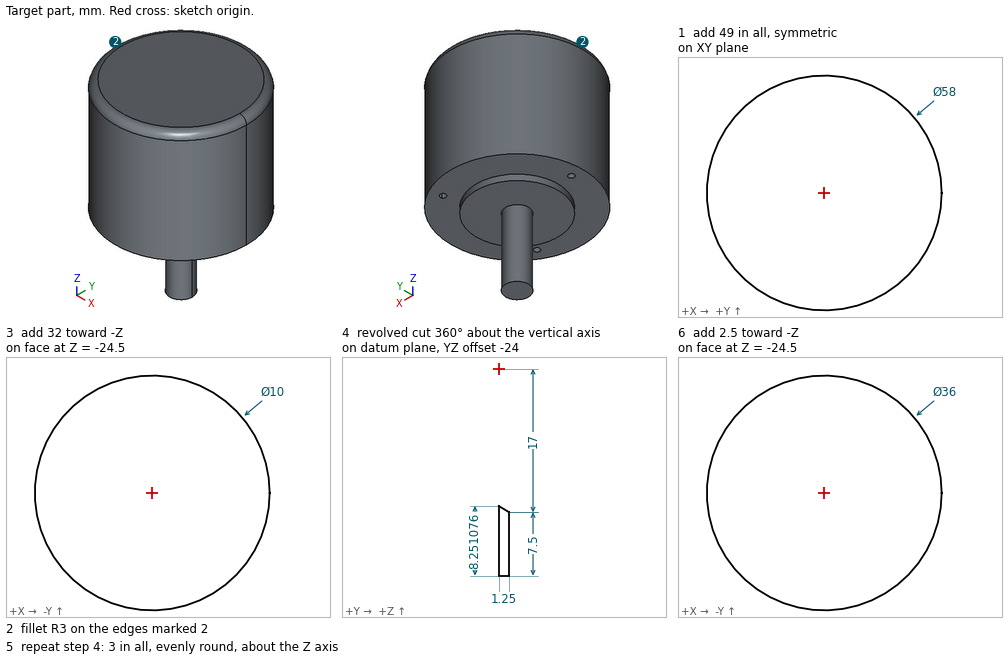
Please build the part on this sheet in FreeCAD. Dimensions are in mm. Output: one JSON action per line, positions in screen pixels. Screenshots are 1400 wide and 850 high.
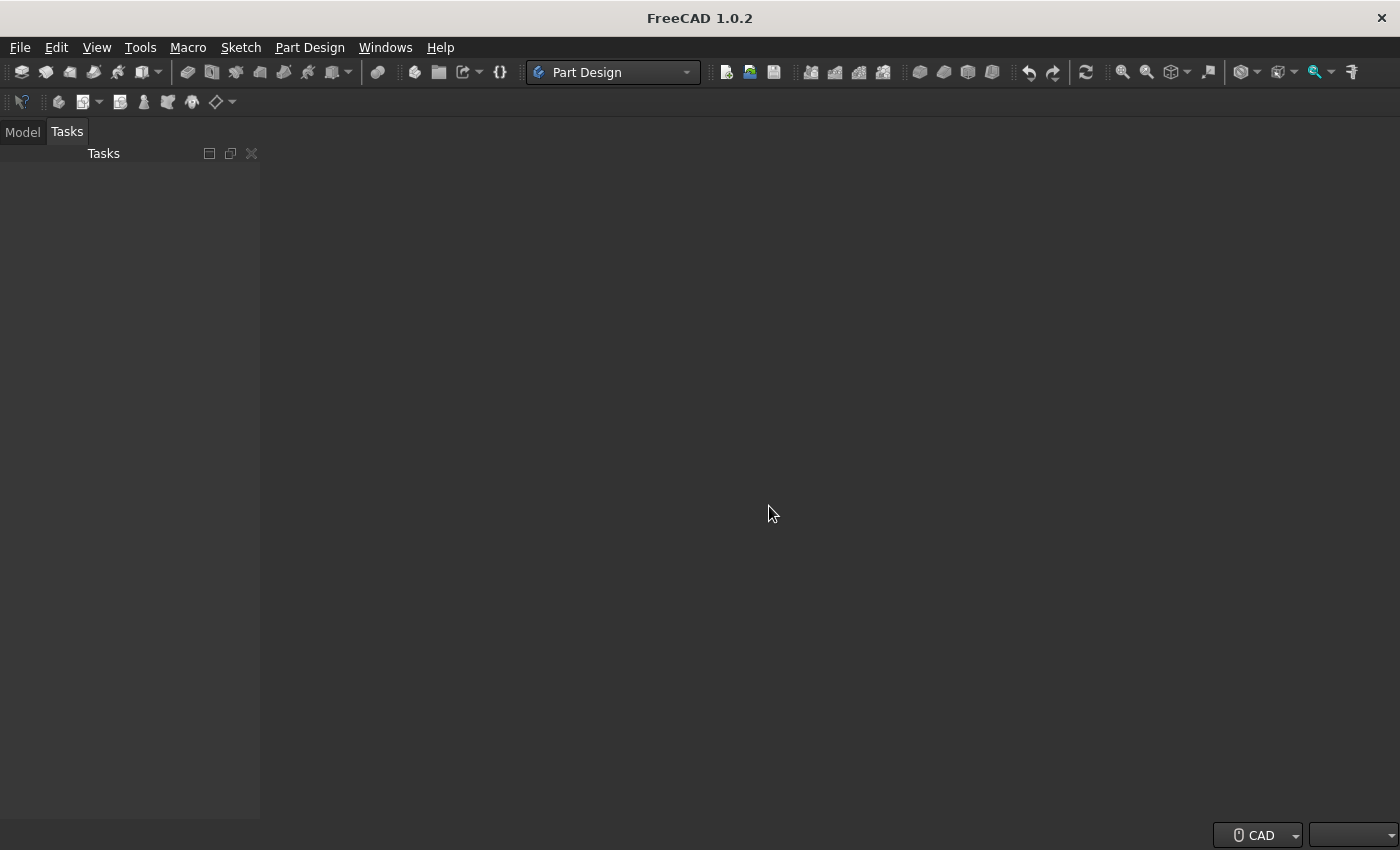
{"action": "left_click", "coordinate": [726, 72]}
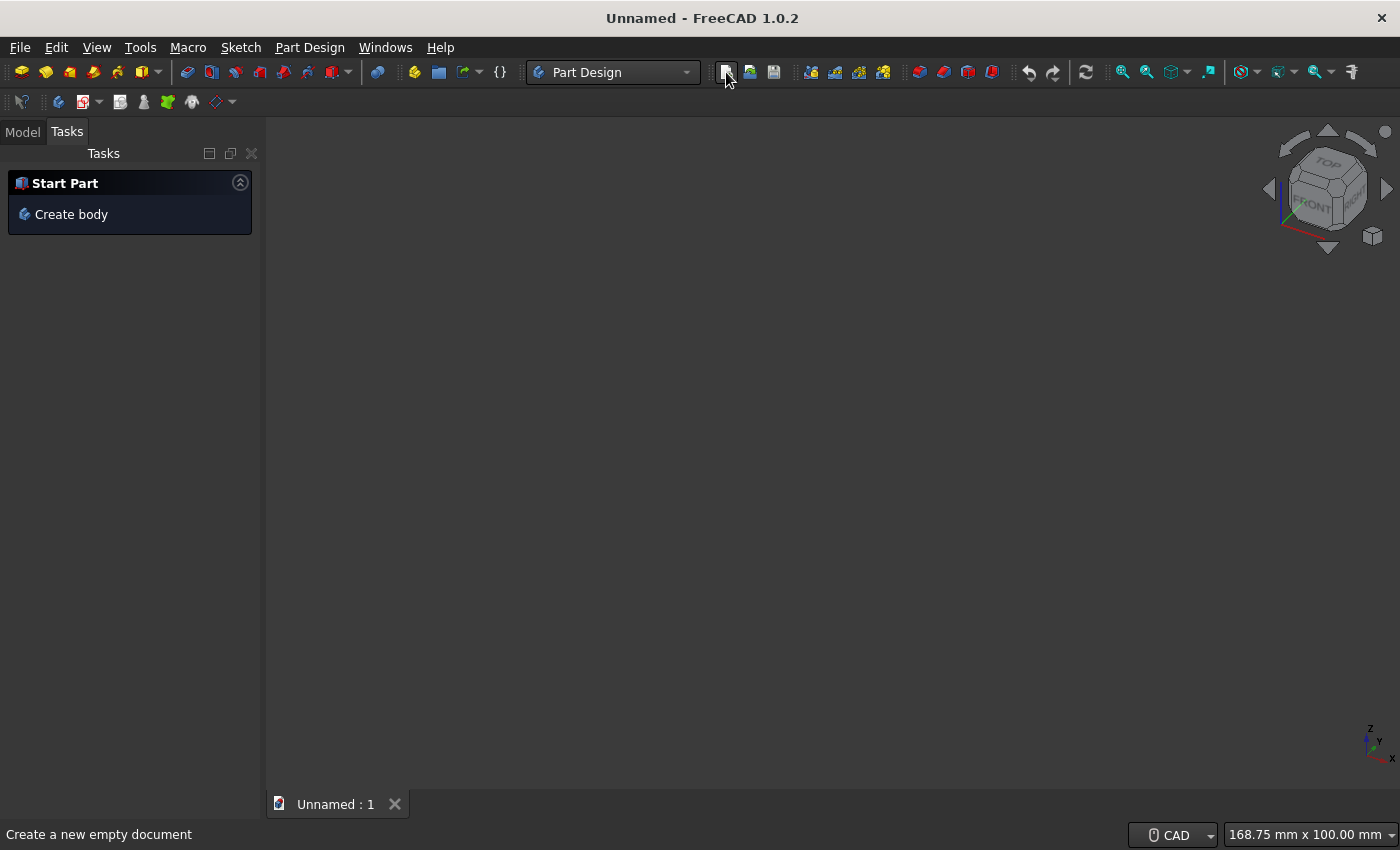
{"action": "left_click", "coordinate": [84, 102]}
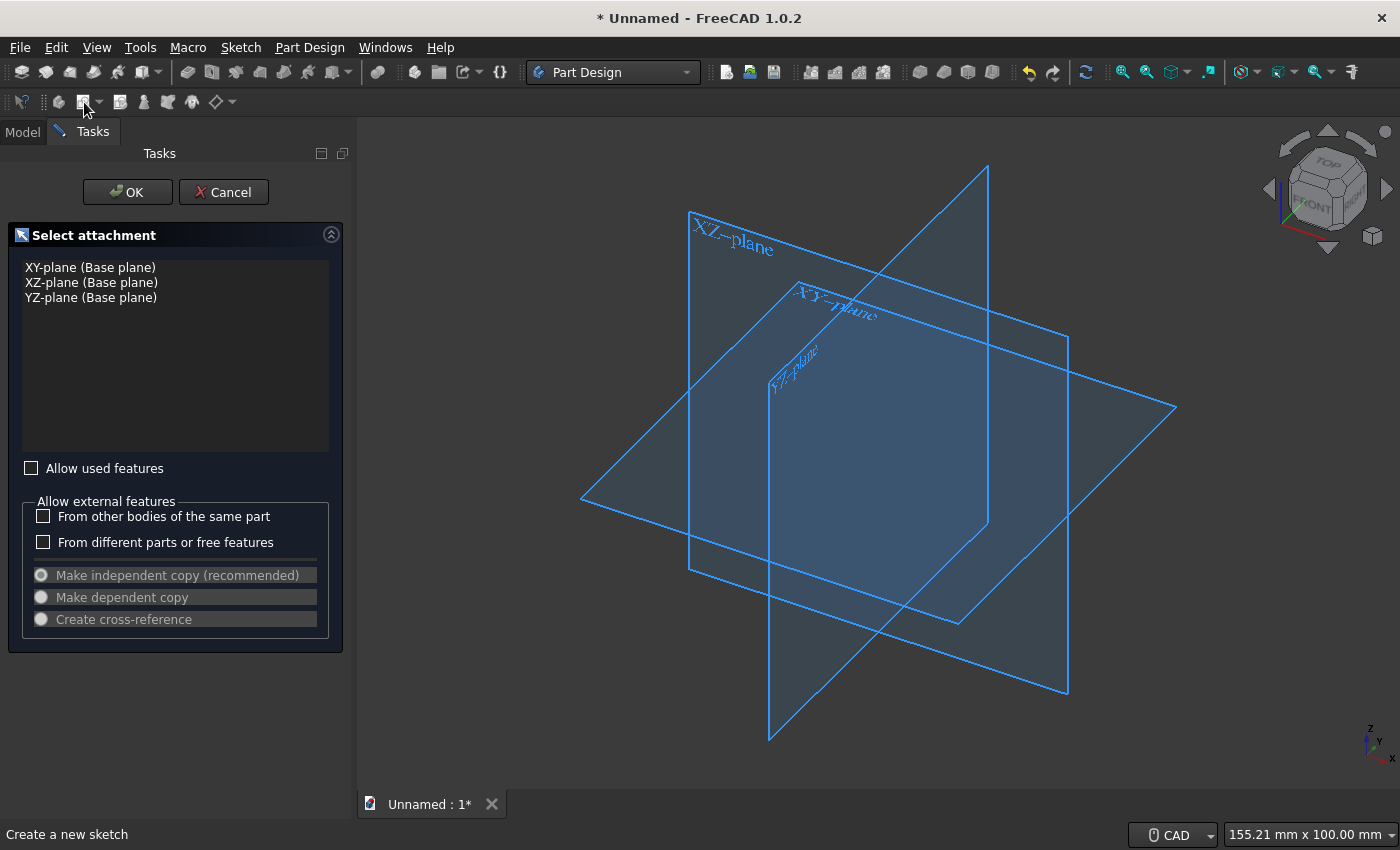
{"action": "left_click", "coordinate": [82, 268]}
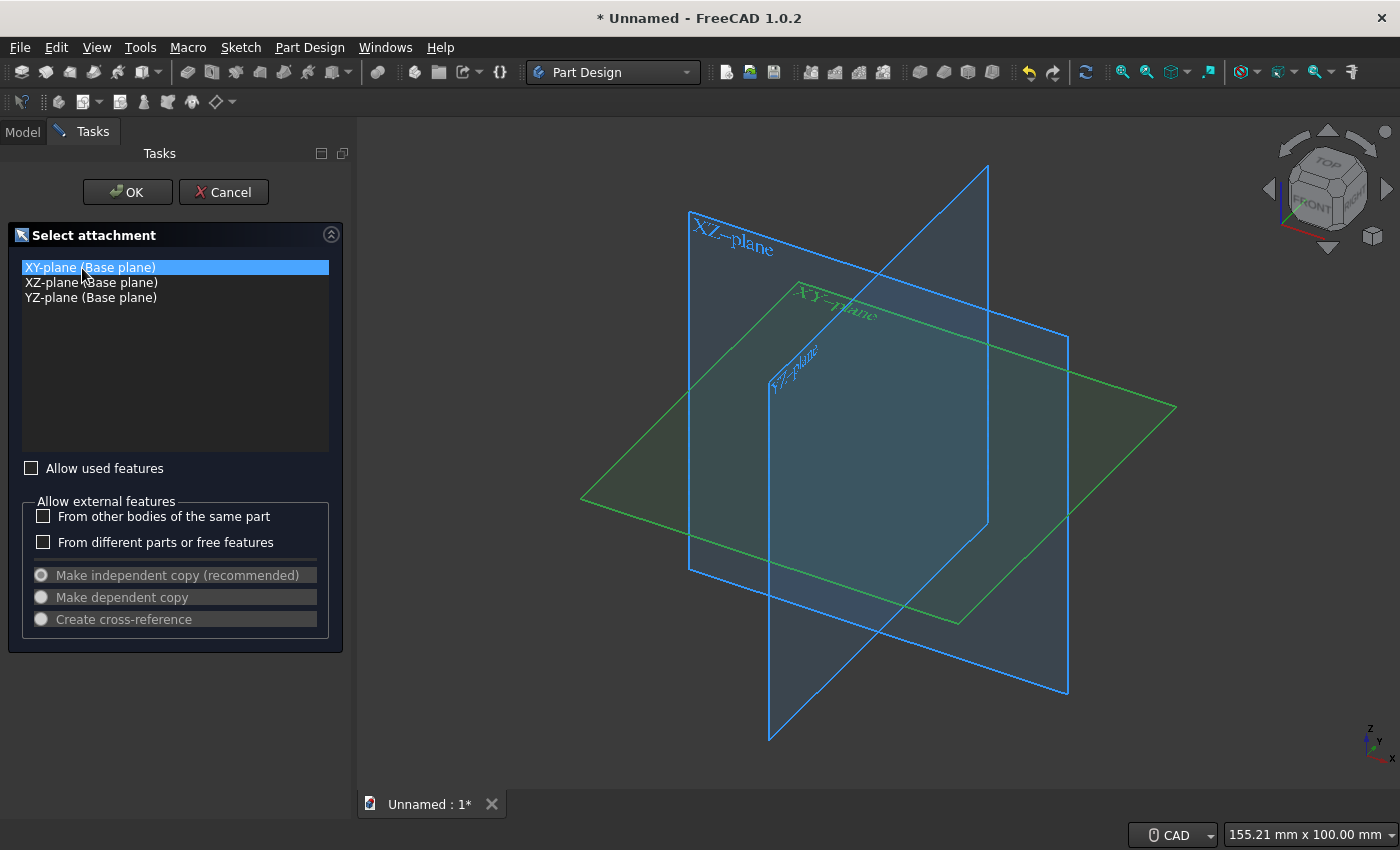
{"action": "left_click", "coordinate": [128, 192]}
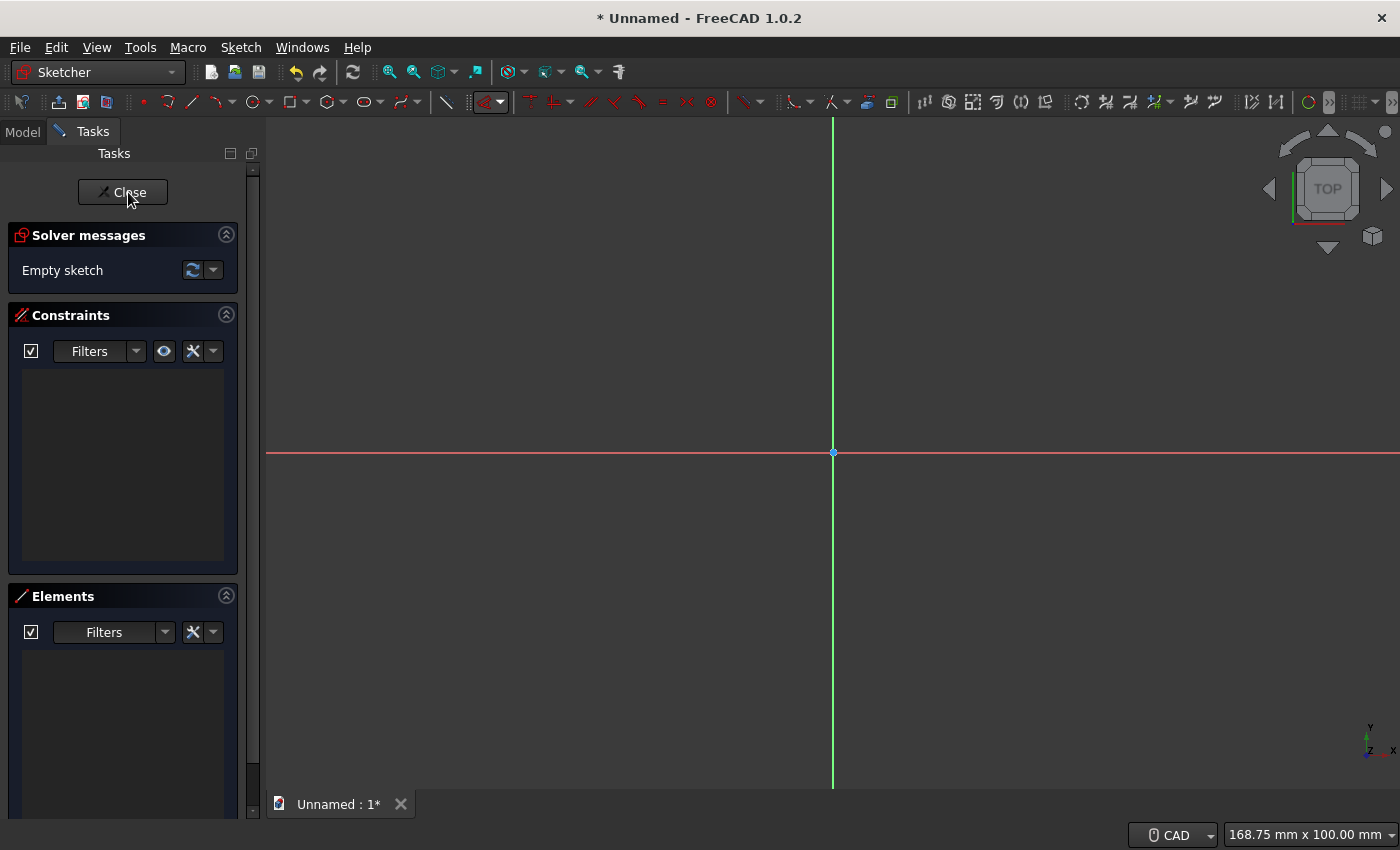
{"action": "left_click", "coordinate": [254, 102]}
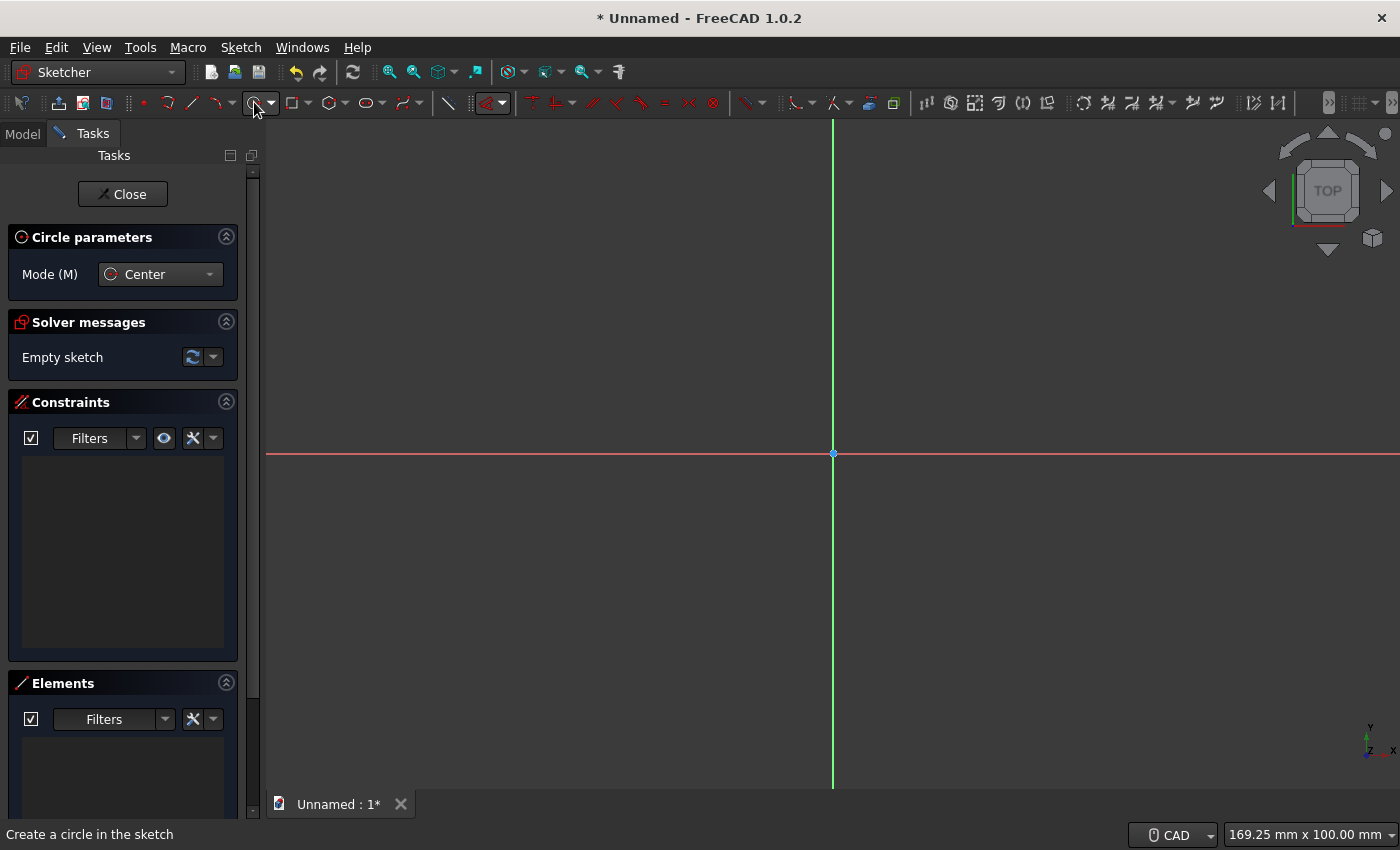
{"action": "left_click", "coordinate": [833, 454]}
{"action": "left_click", "coordinate": [970, 317]}
{"action": "key", "text": "Escape"}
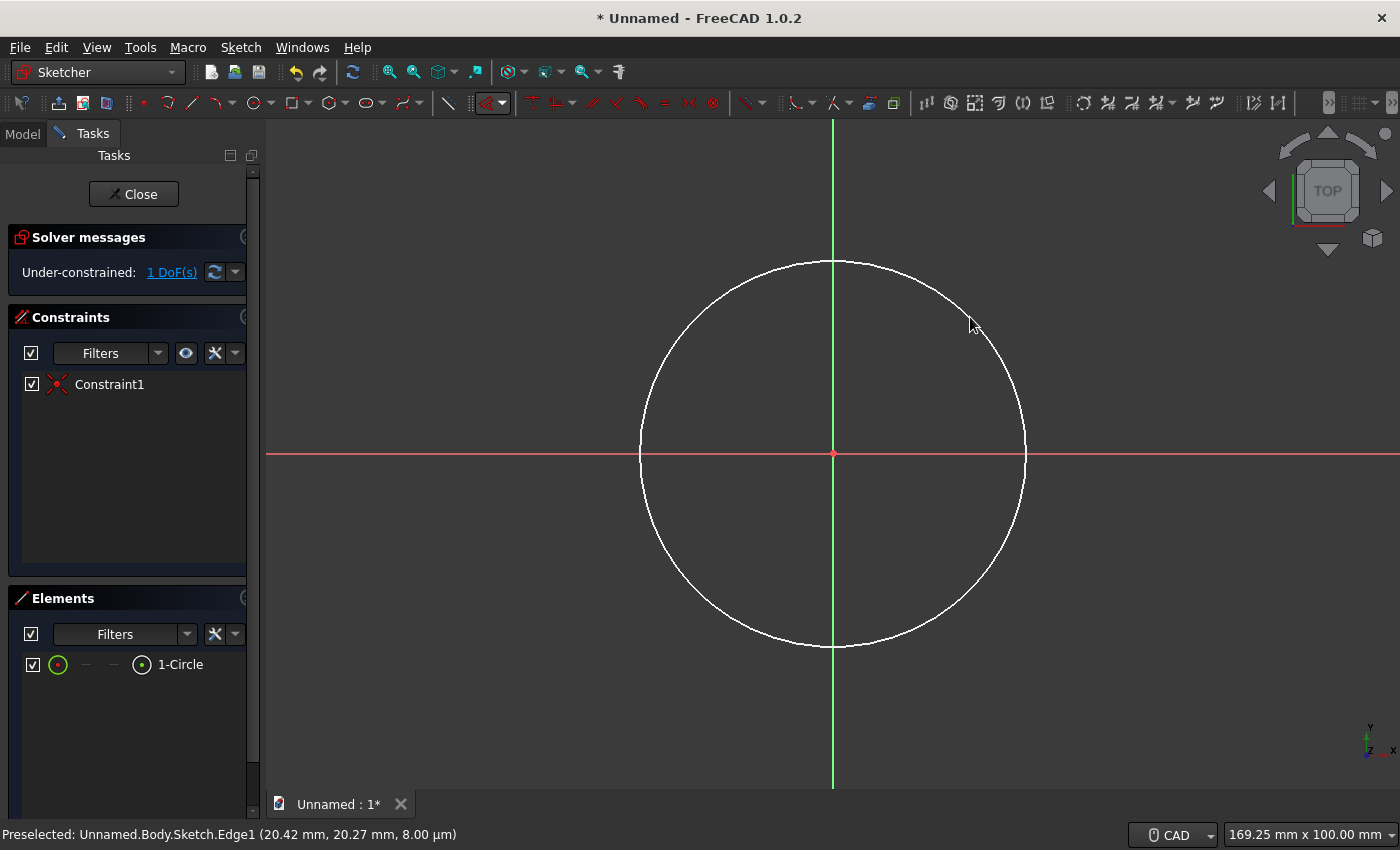
{"action": "left_click", "coordinate": [486, 104]}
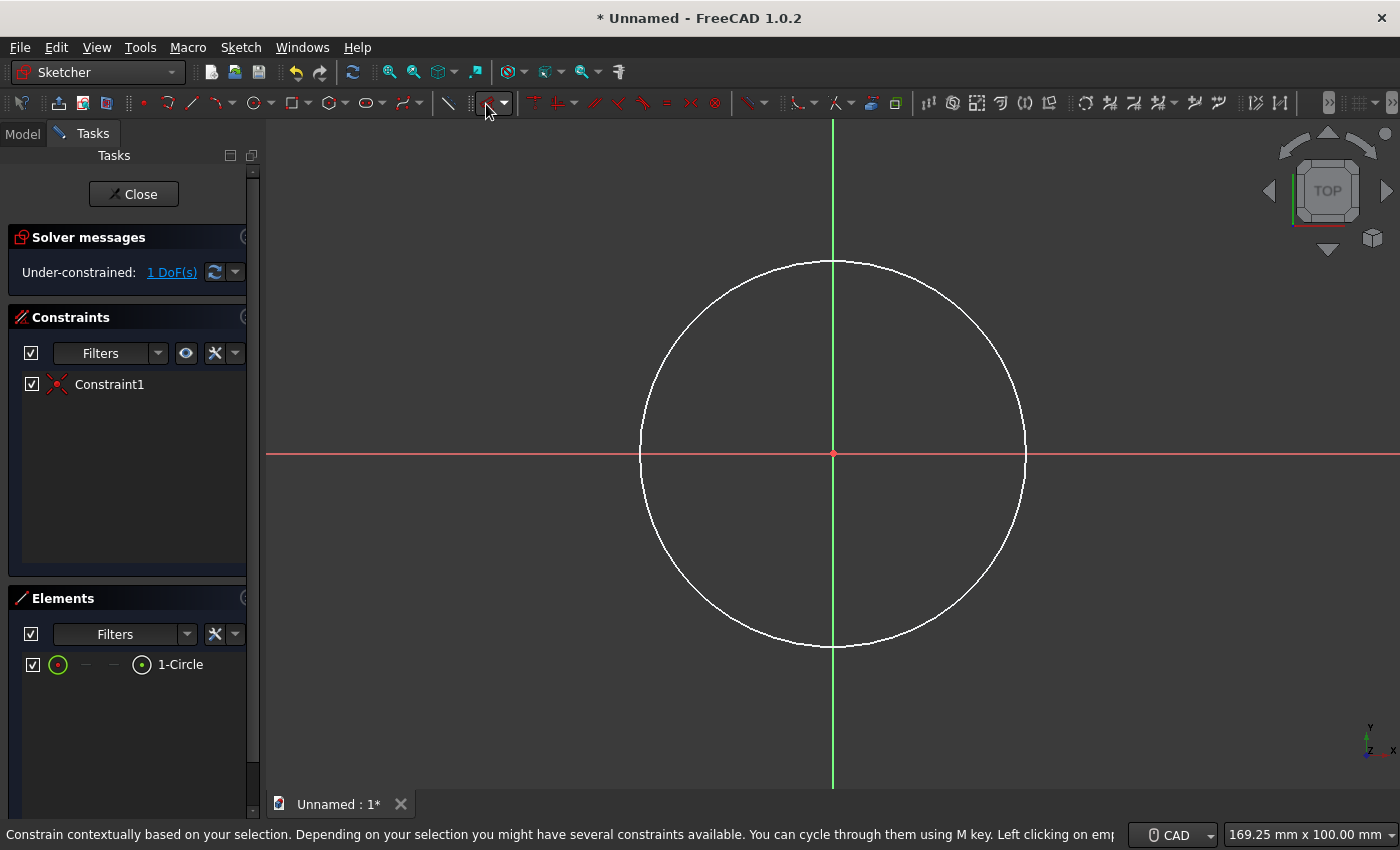
{"action": "left_click", "coordinate": [969, 317]}
{"action": "left_click", "coordinate": [992, 294]}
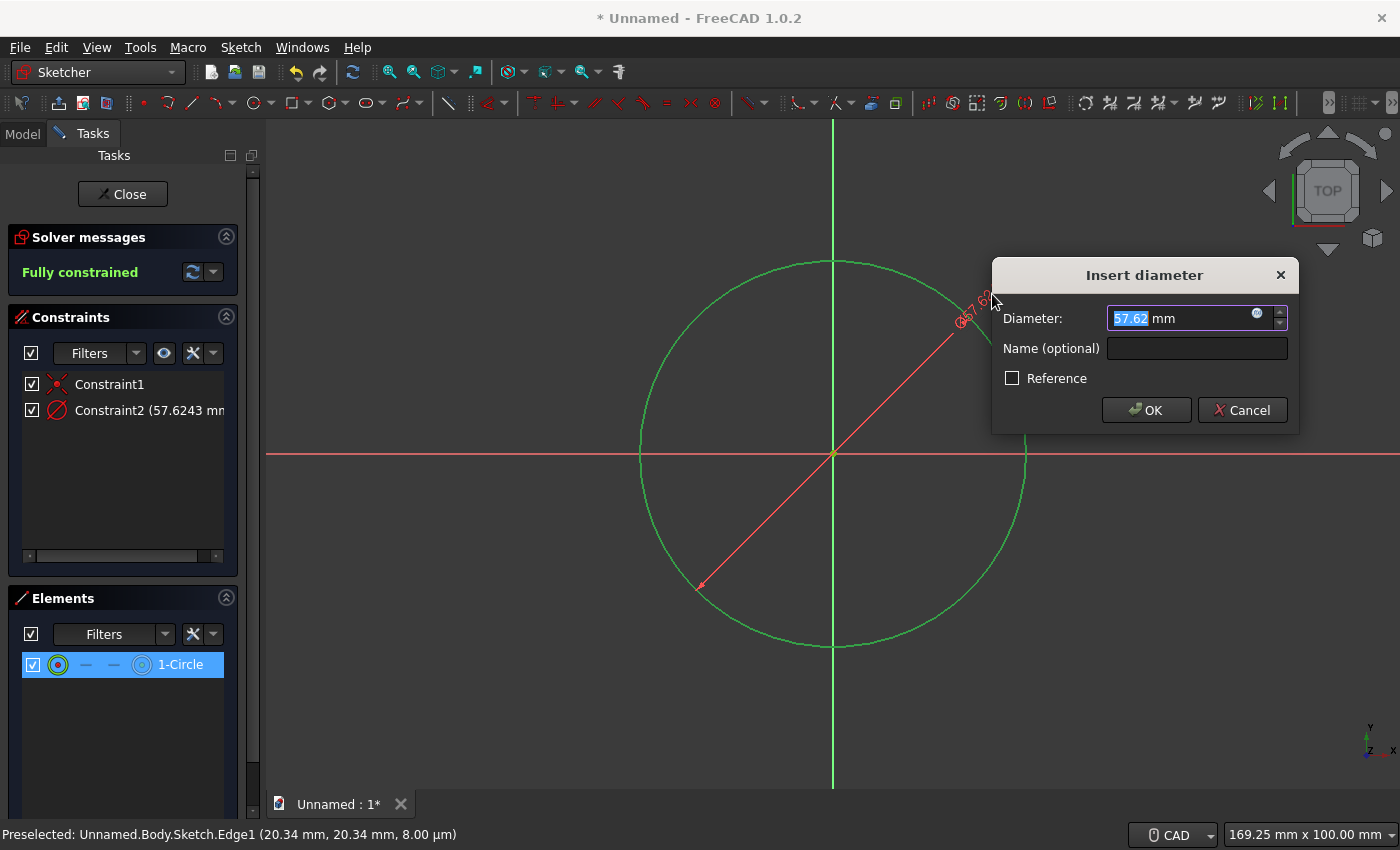
{"action": "type", "text": "58"}
{"action": "key", "text": "Return"}
{"action": "key", "text": "Escape"}